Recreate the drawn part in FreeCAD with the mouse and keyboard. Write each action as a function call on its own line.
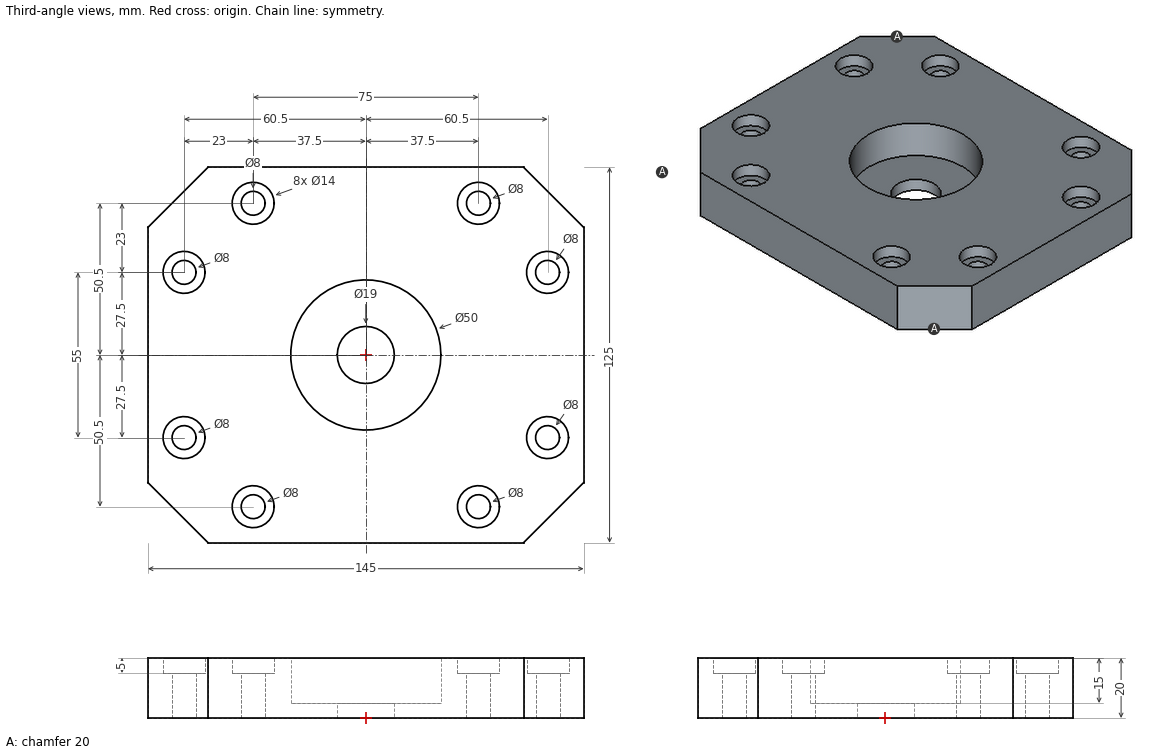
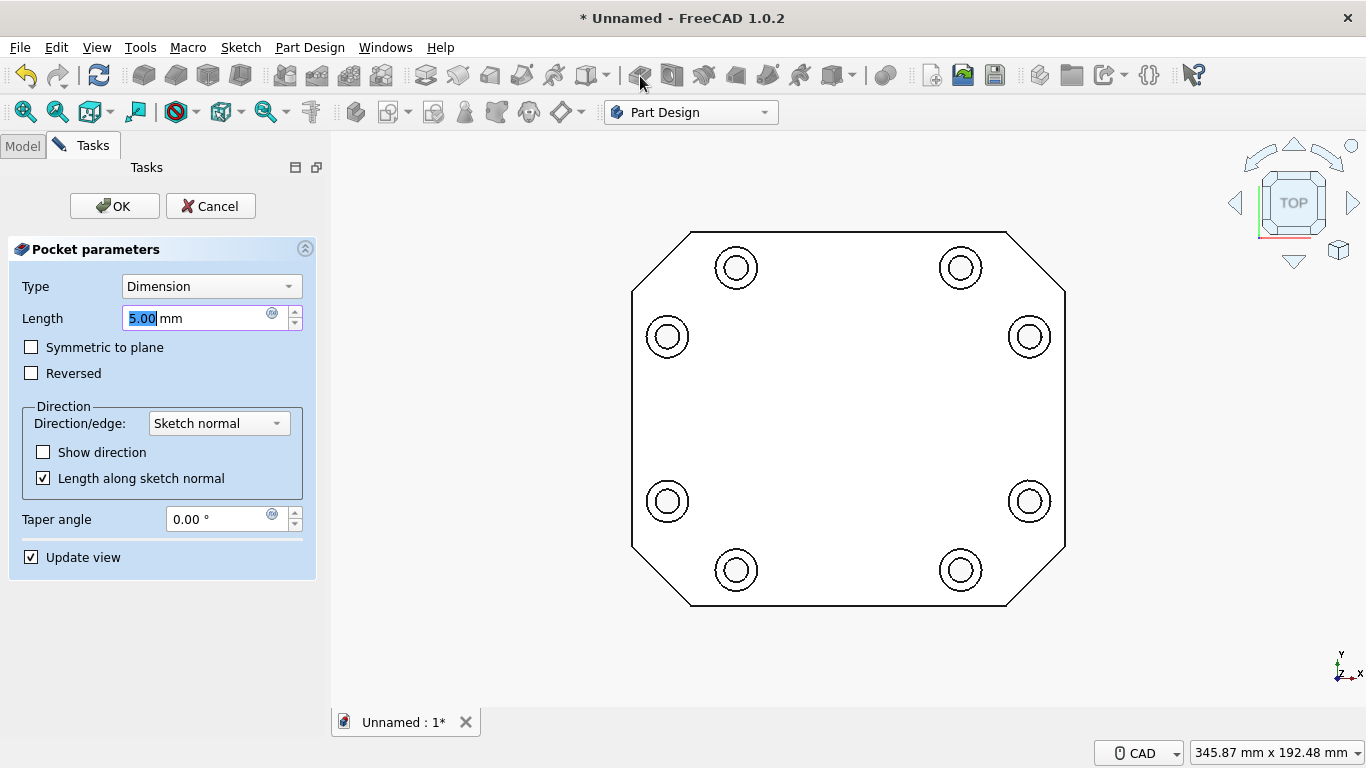
click(212, 286)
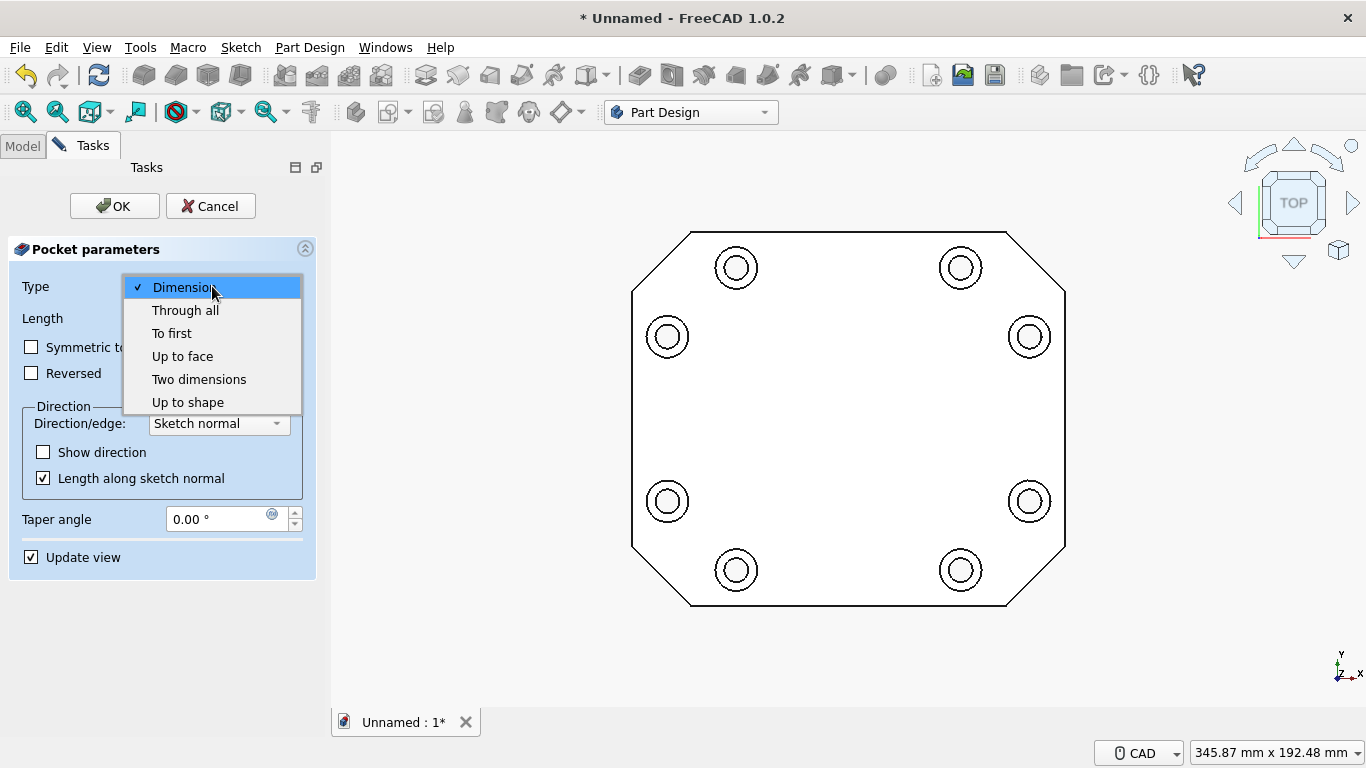
click(212, 334)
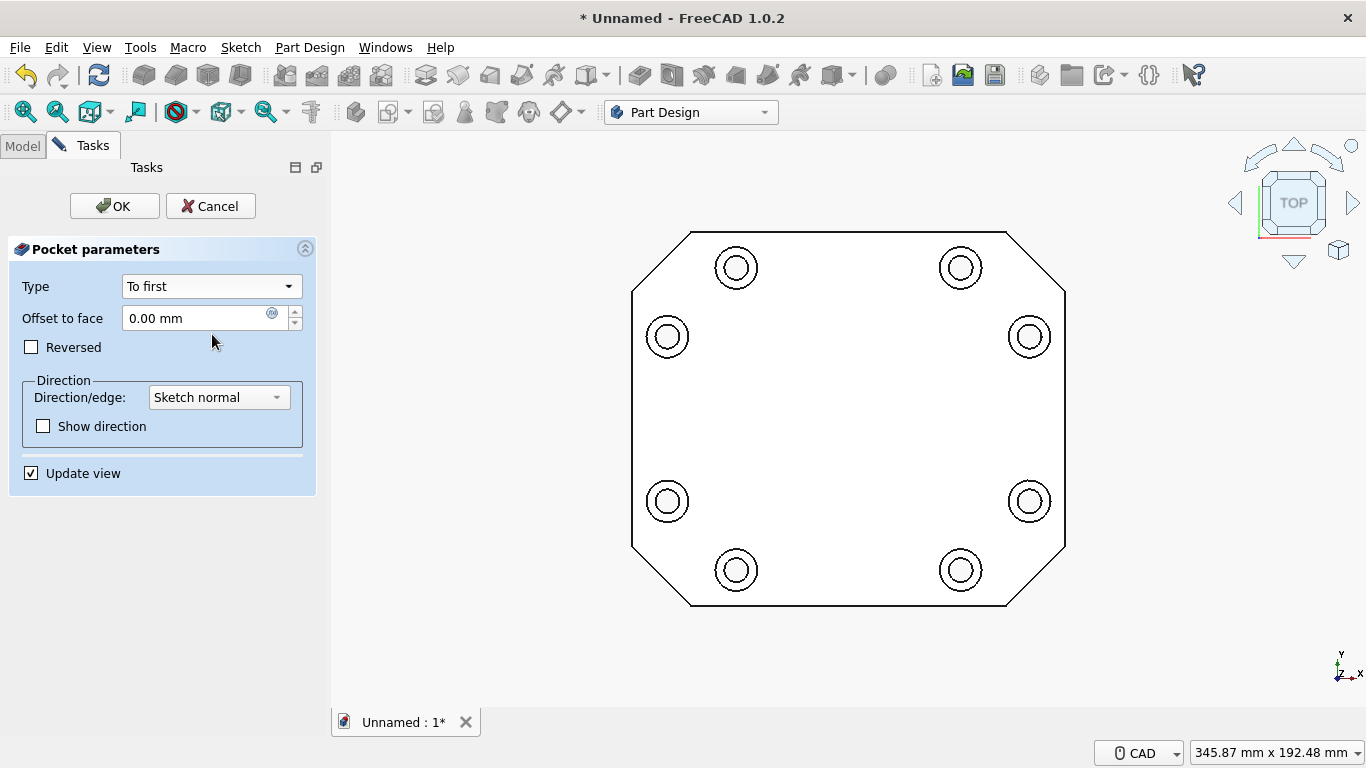
click(30, 347)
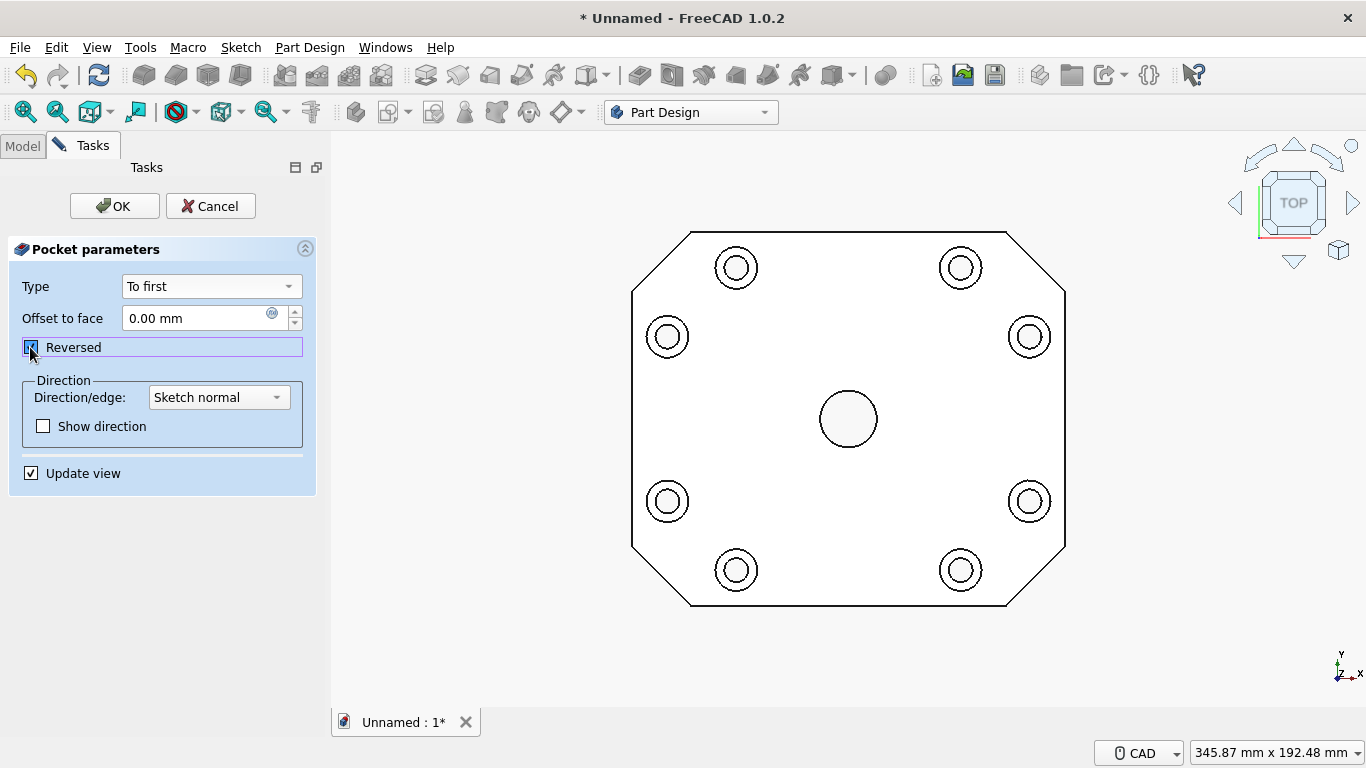
click(115, 206)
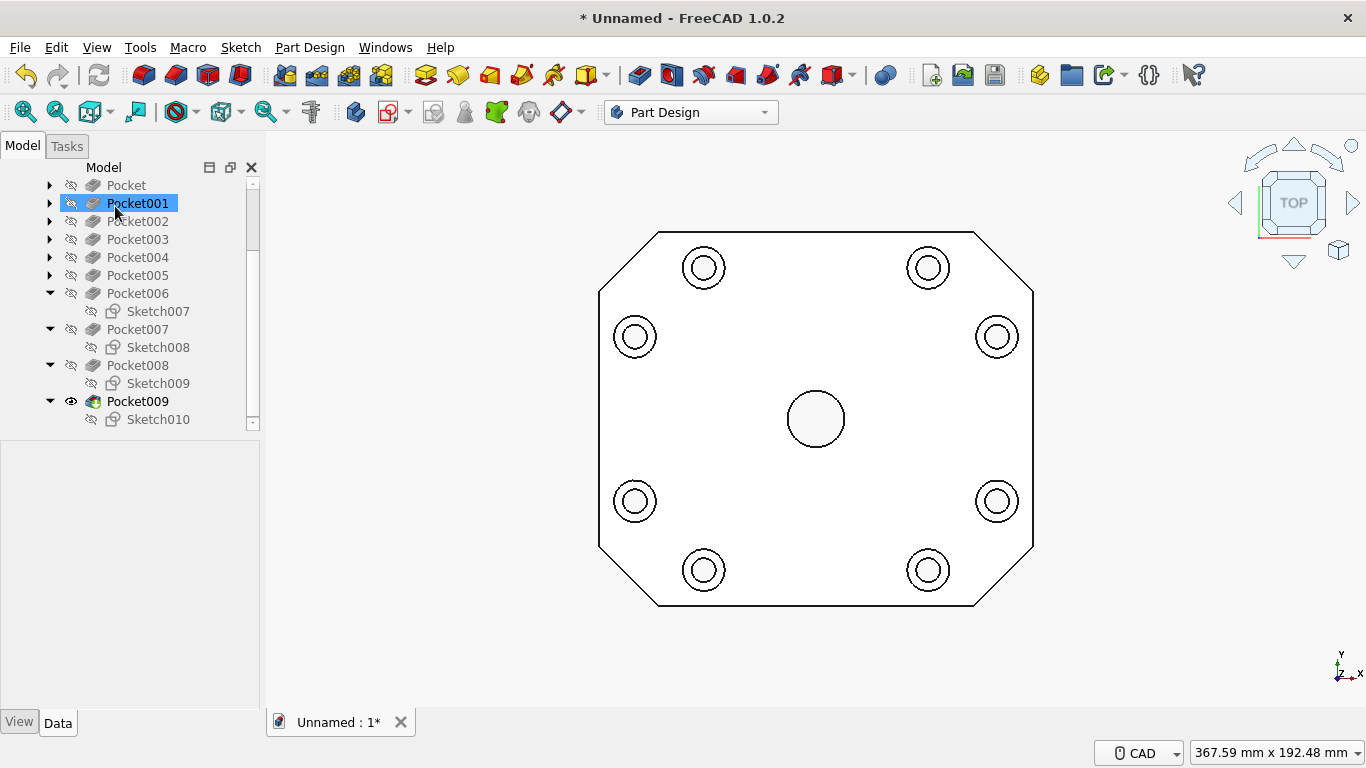
click(940, 418)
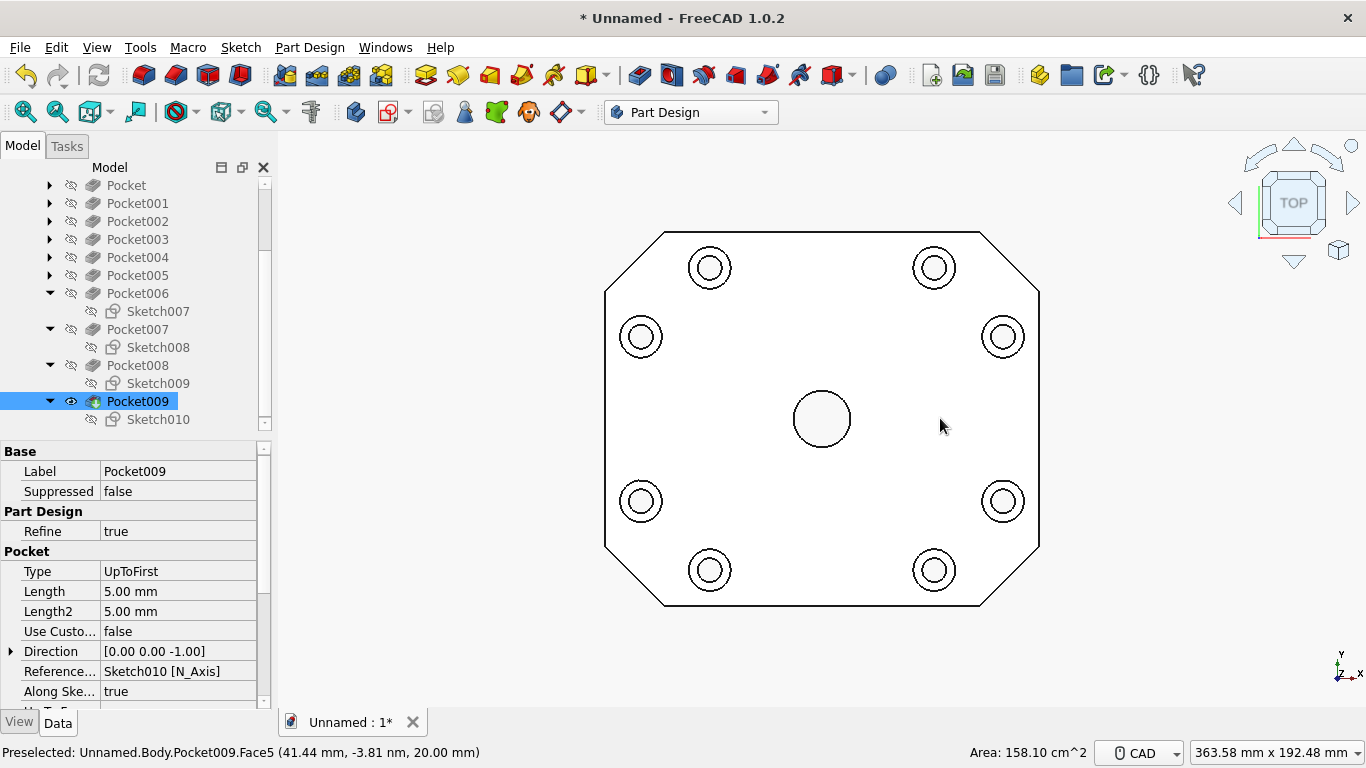
click(388, 112)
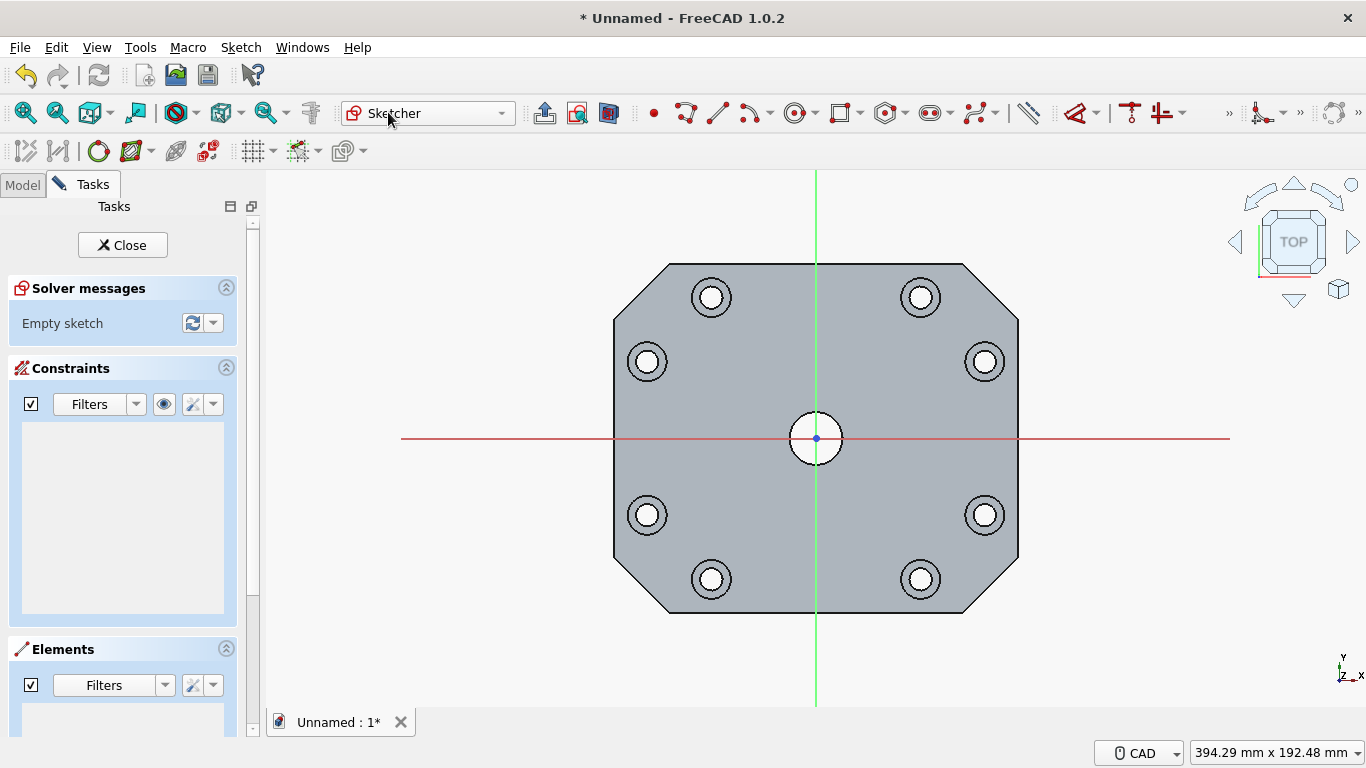
scroll(872, 438, up, 4)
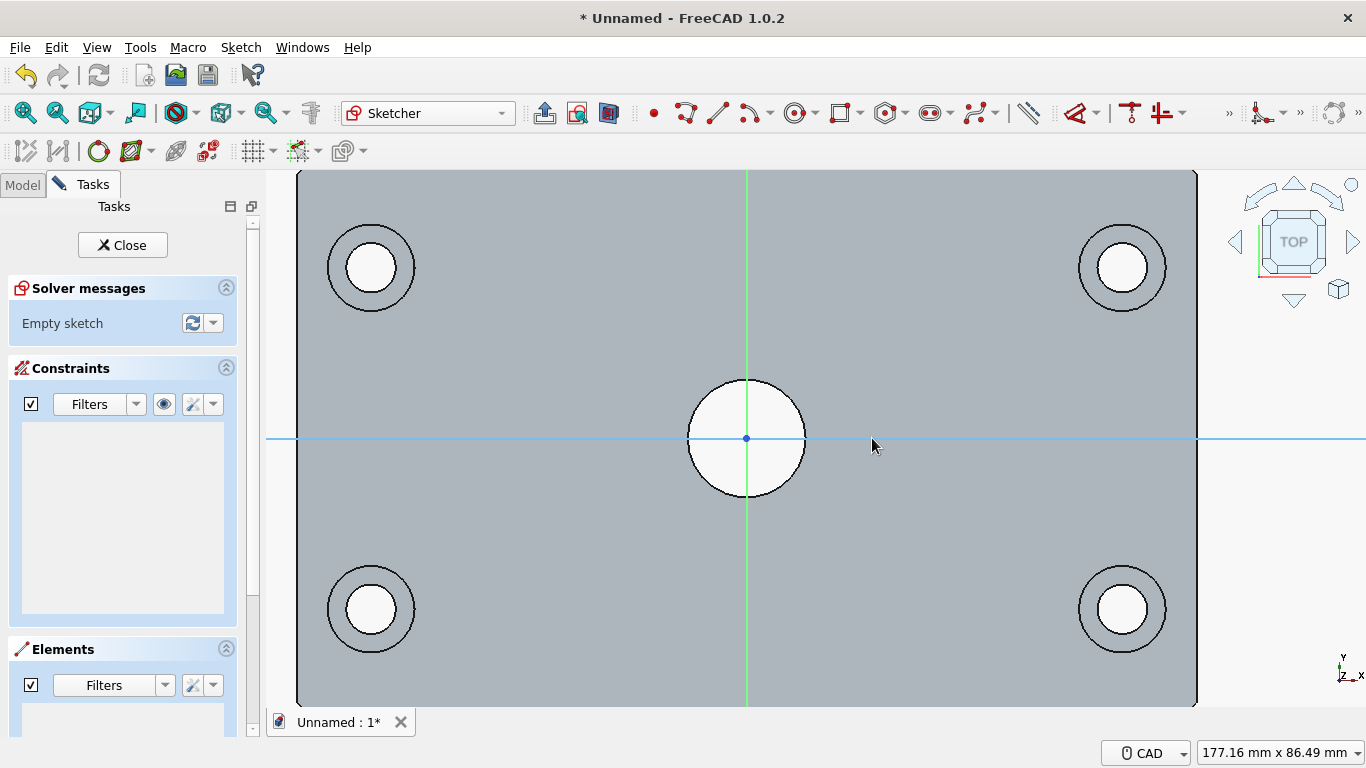
click(796, 114)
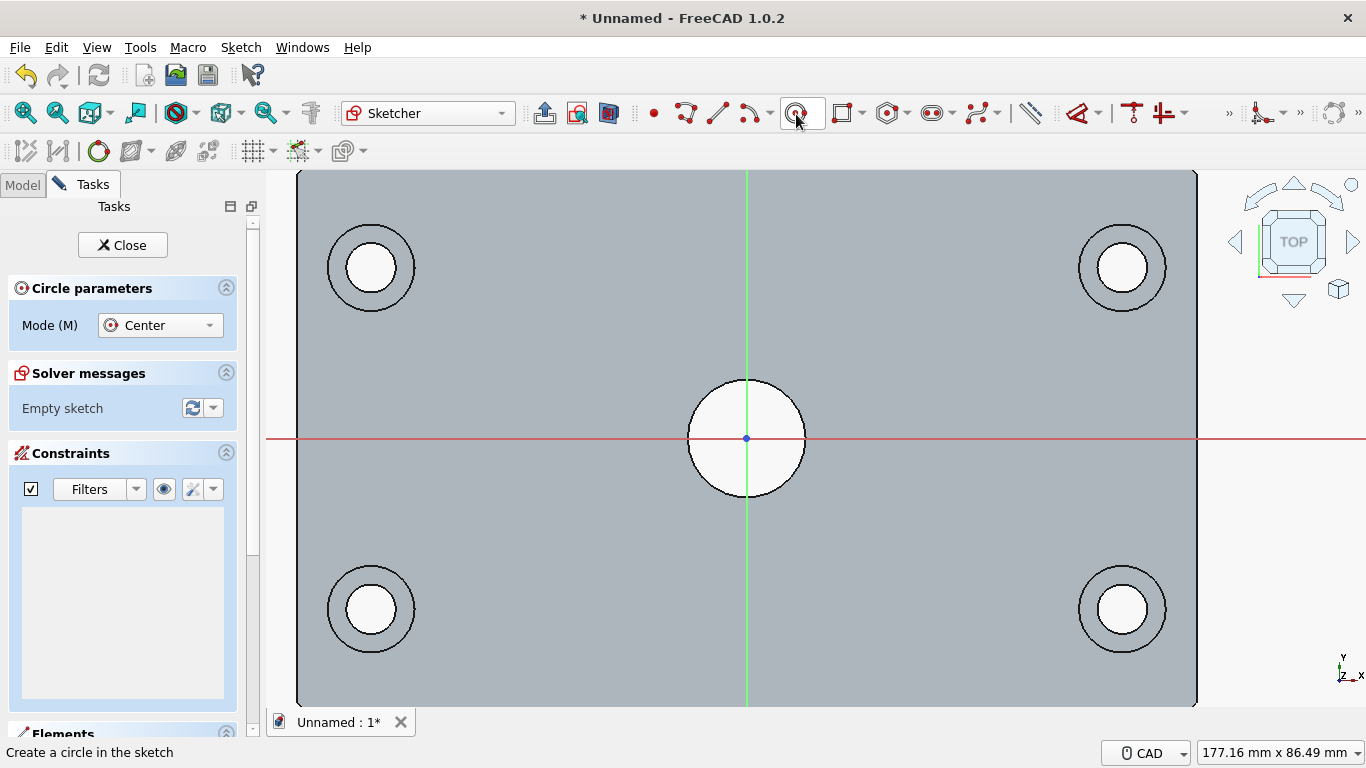
click(747, 438)
click(856, 329)
key(Escape)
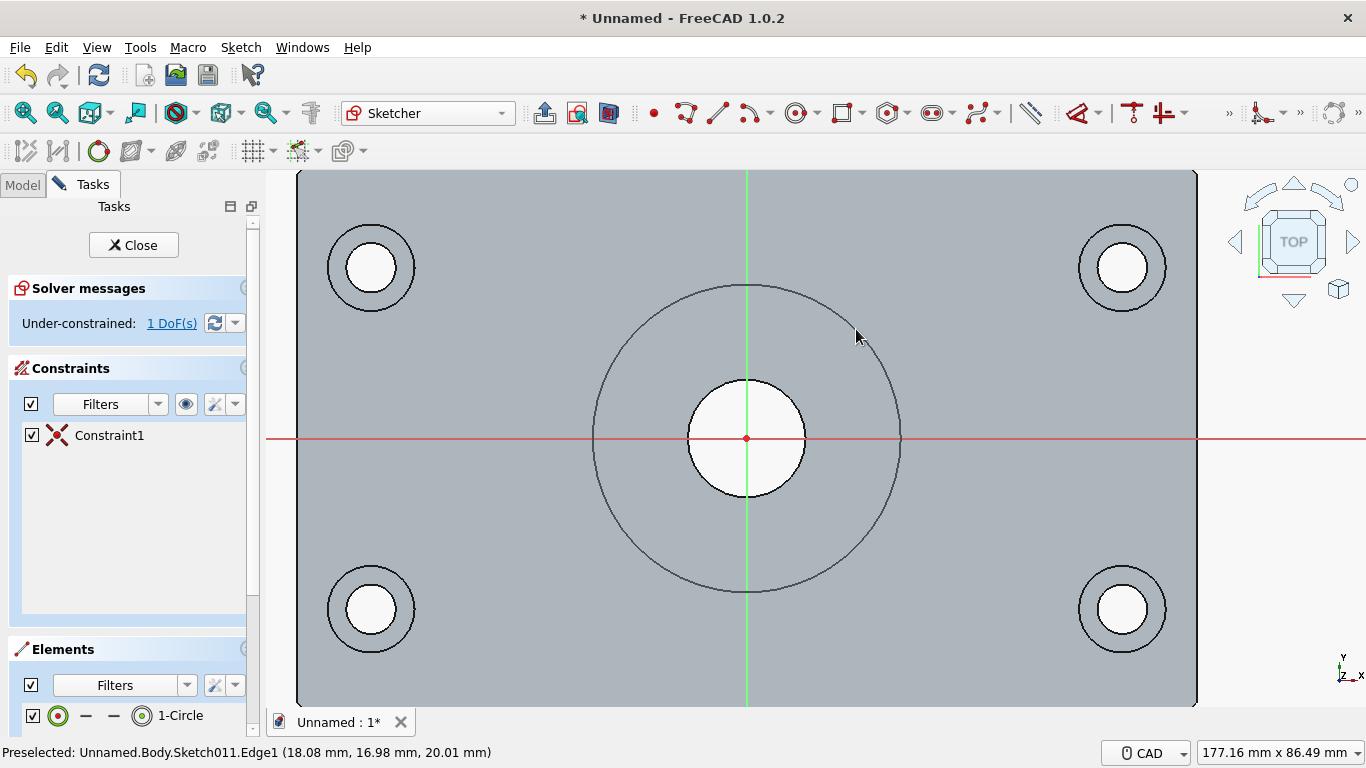
key(d)